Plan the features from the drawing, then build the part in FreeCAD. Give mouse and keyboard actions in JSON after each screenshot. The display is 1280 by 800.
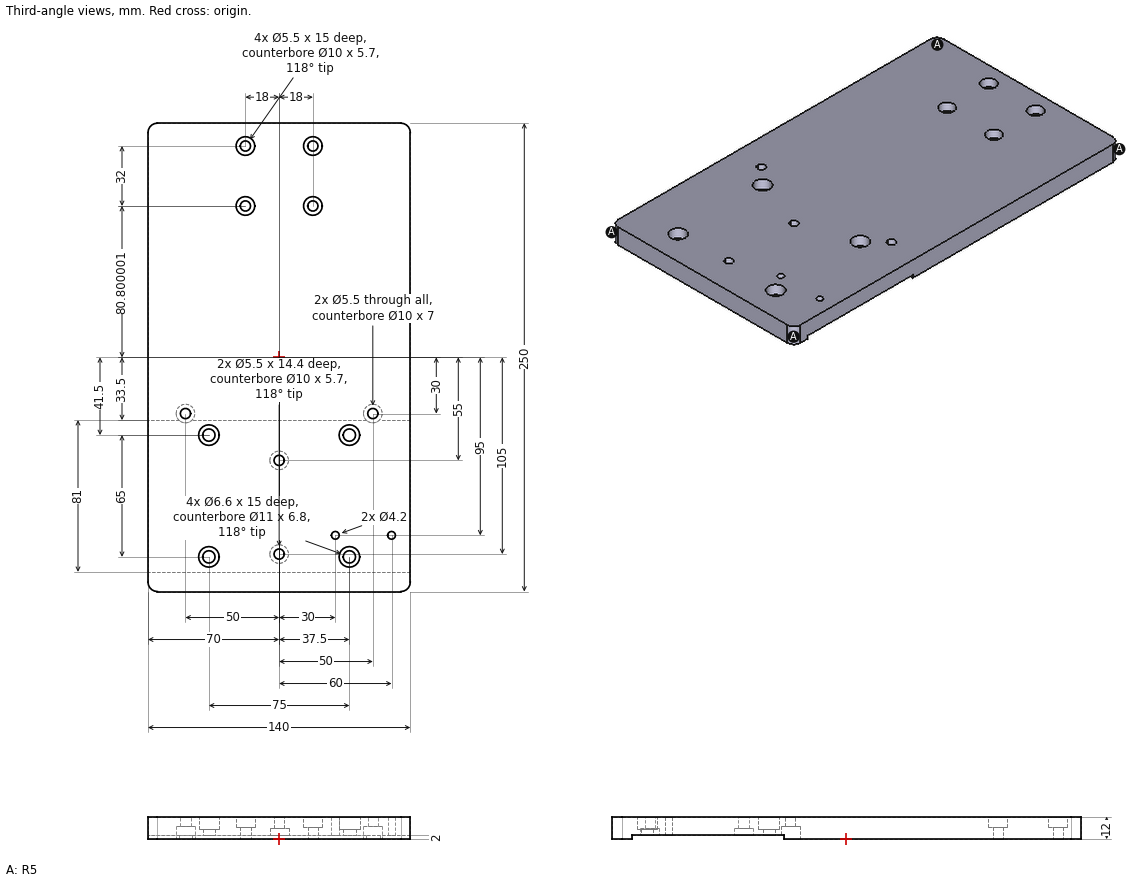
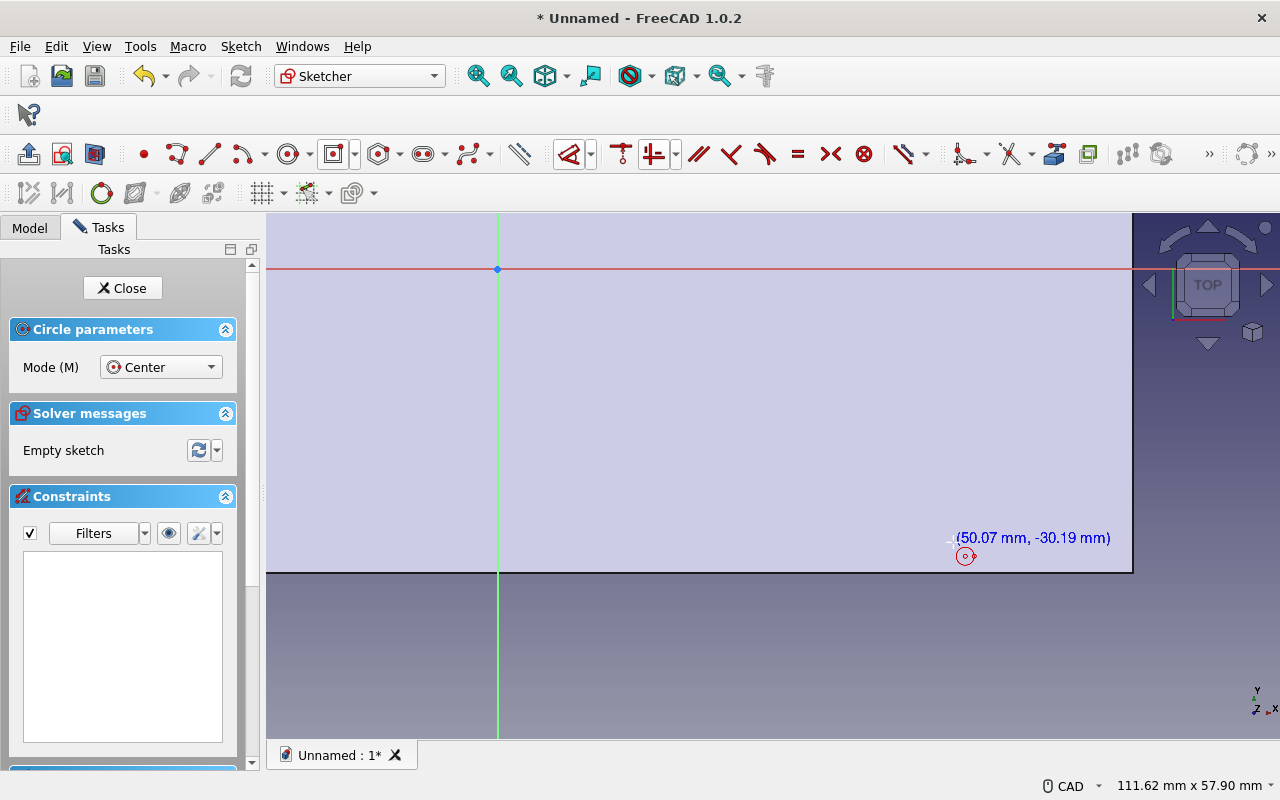
{"action": "left_click", "coordinate": [952, 542]}
{"action": "left_click", "coordinate": [969, 524]}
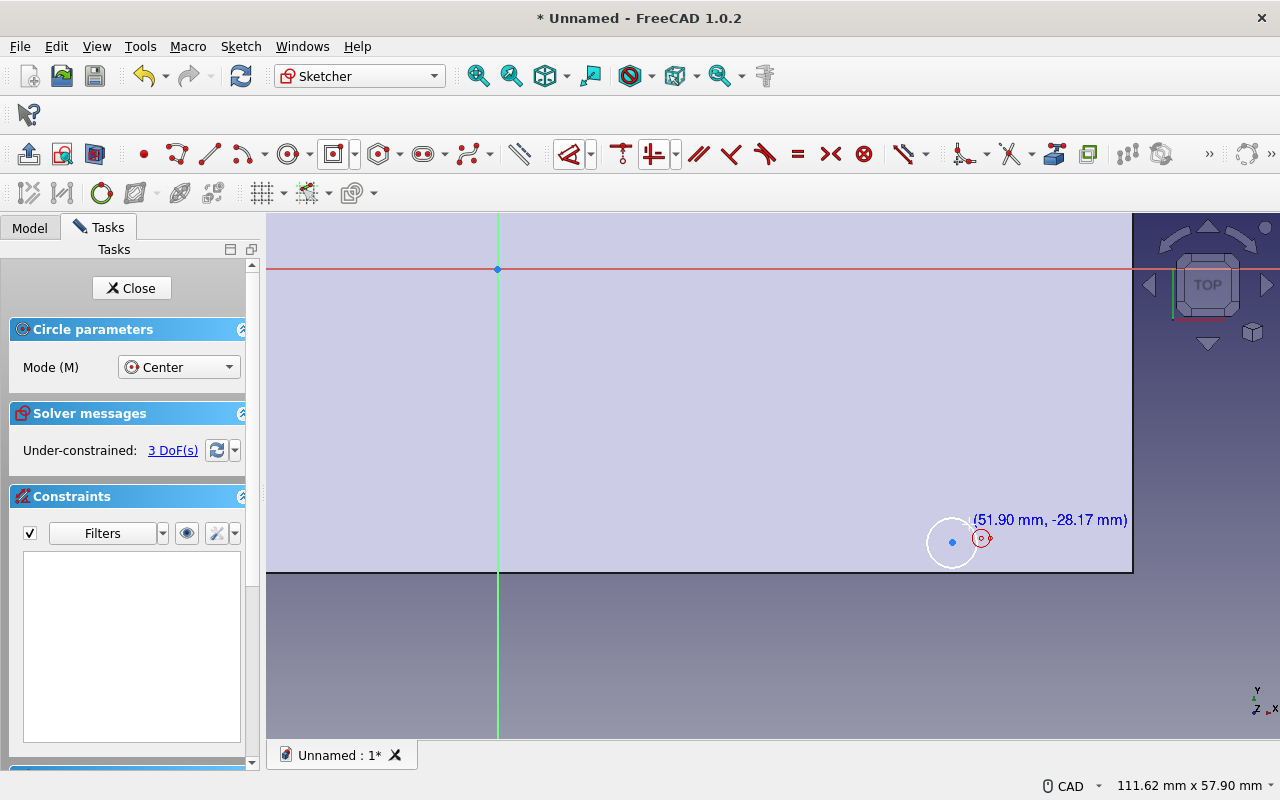
{"action": "scroll", "coordinate": [956, 547], "scroll_direction": "down", "scroll_amount": 3}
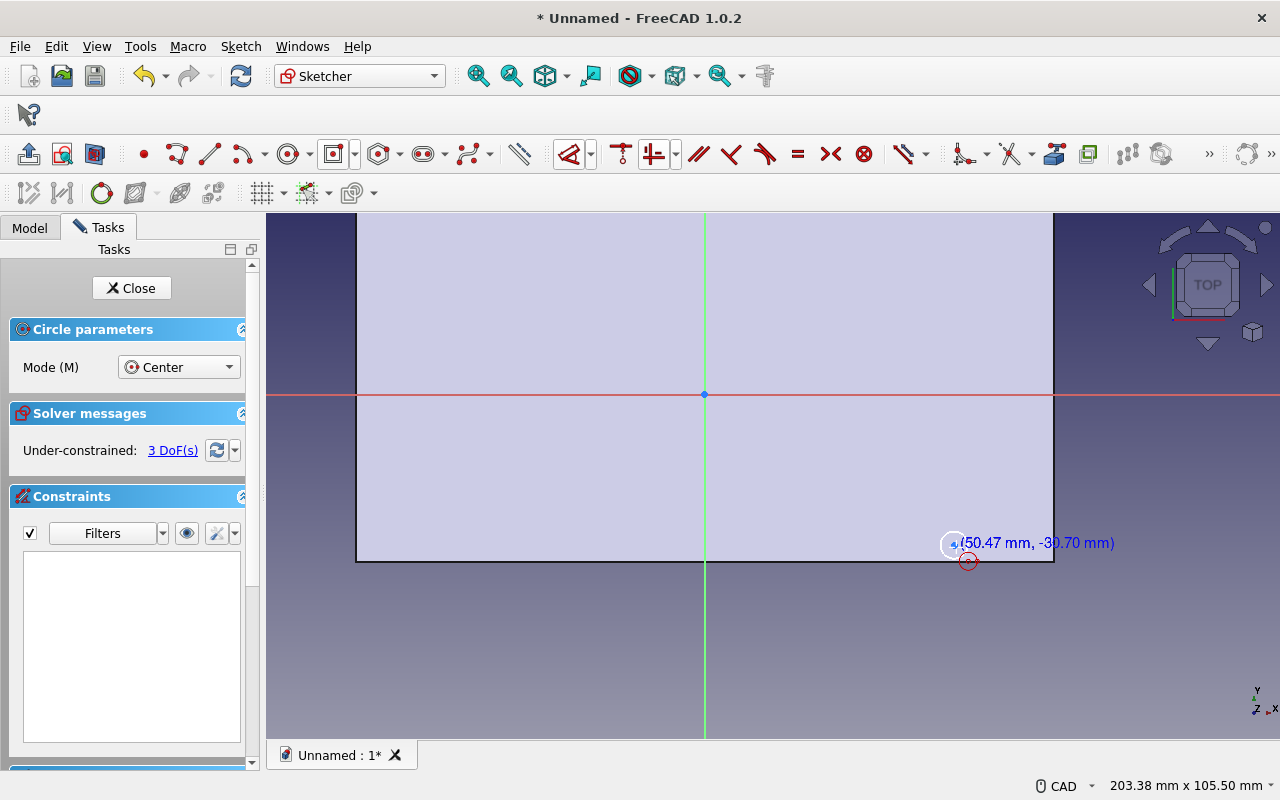
{"action": "scroll", "coordinate": [455, 544], "scroll_direction": "up", "scroll_amount": 3}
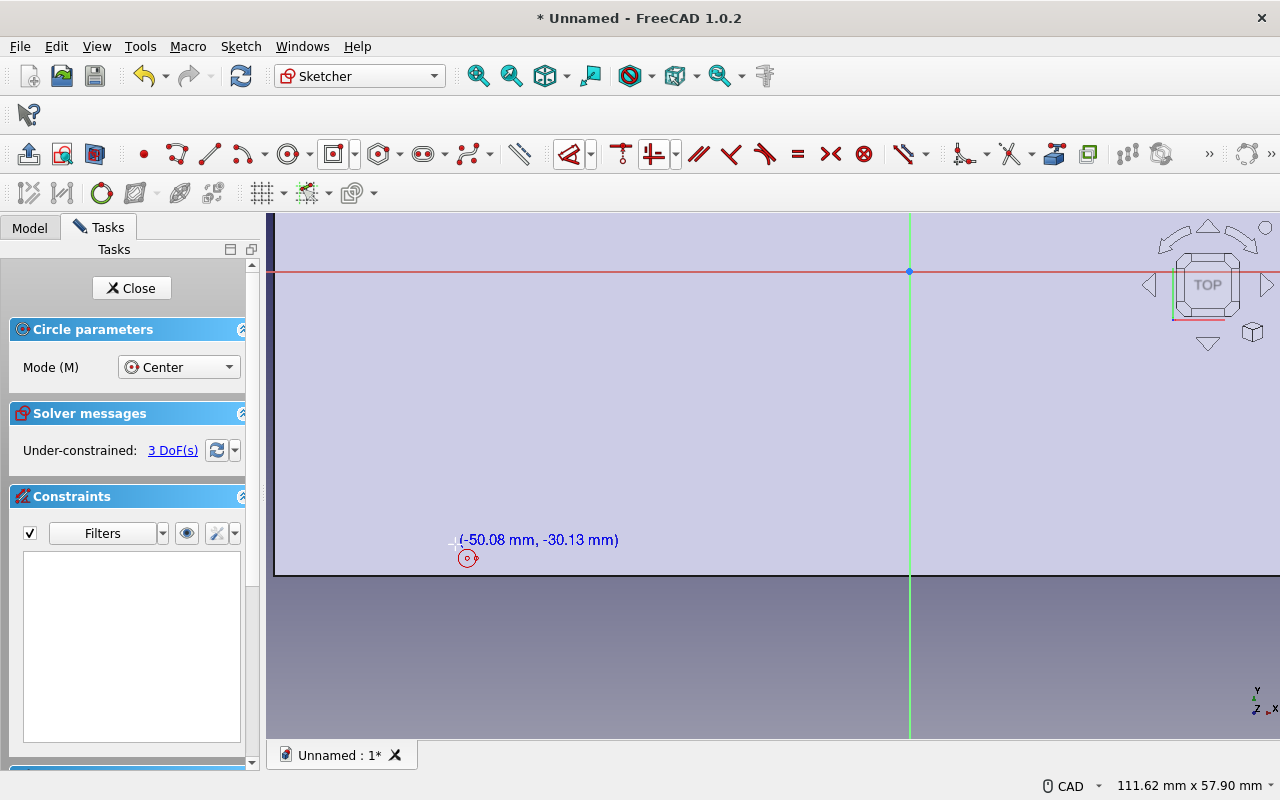
{"action": "left_click", "coordinate": [456, 544]}
{"action": "left_click", "coordinate": [473, 526]}
{"action": "key", "text": "Escape"}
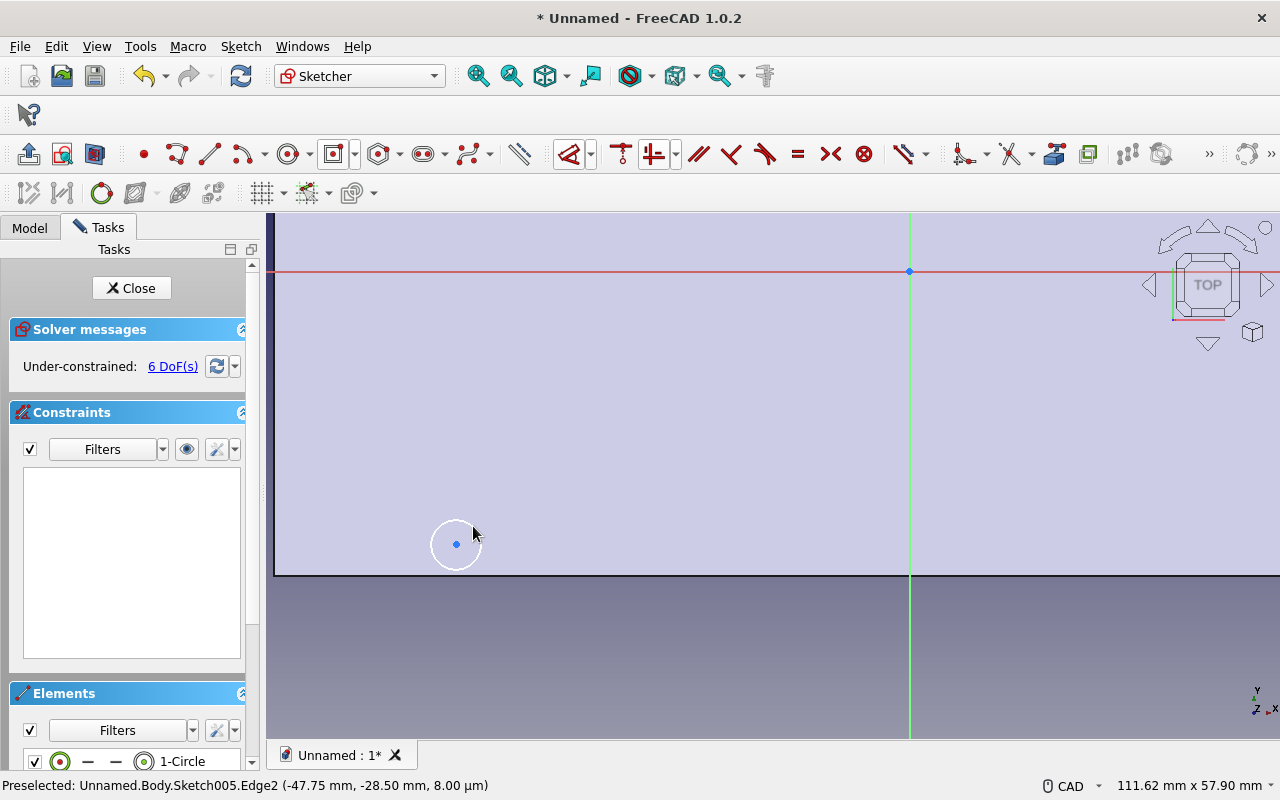
{"action": "scroll", "coordinate": [455, 544], "scroll_direction": "down", "scroll_amount": 3}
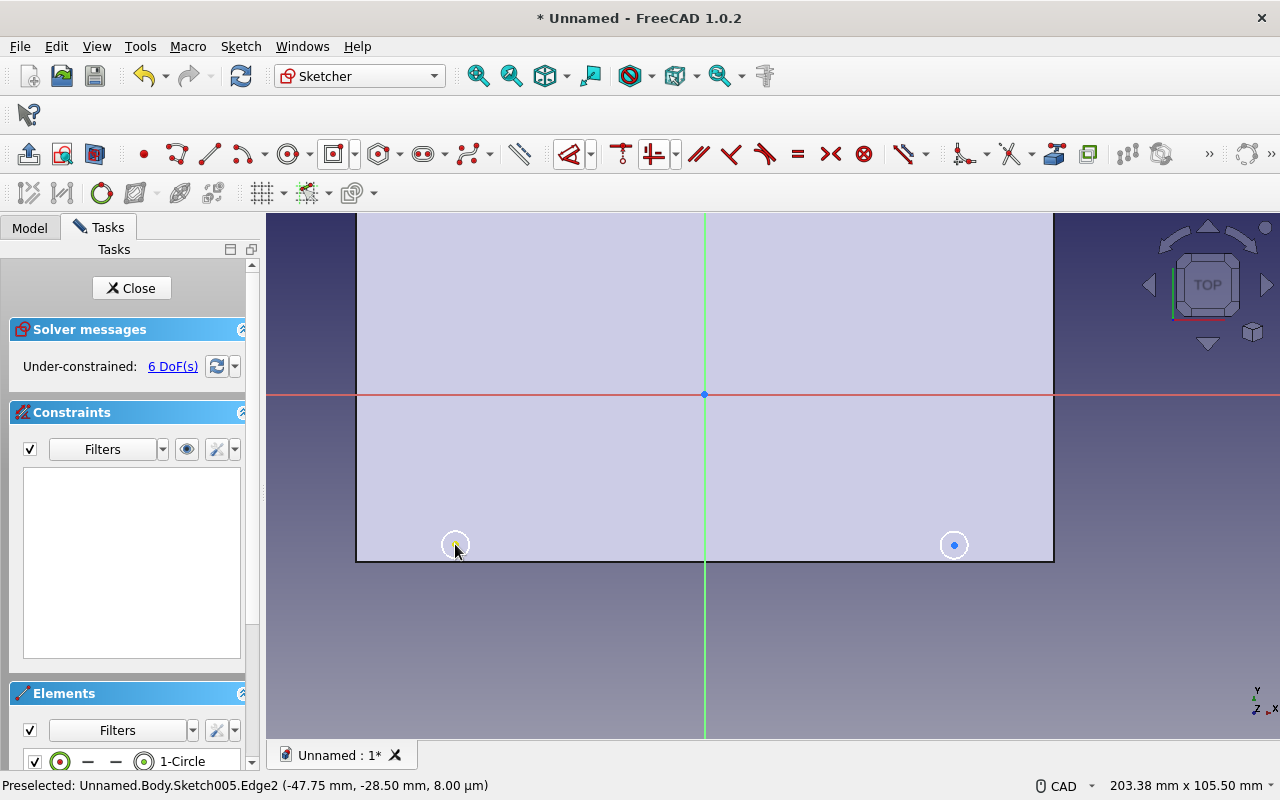
{"action": "left_click", "coordinate": [964, 535]}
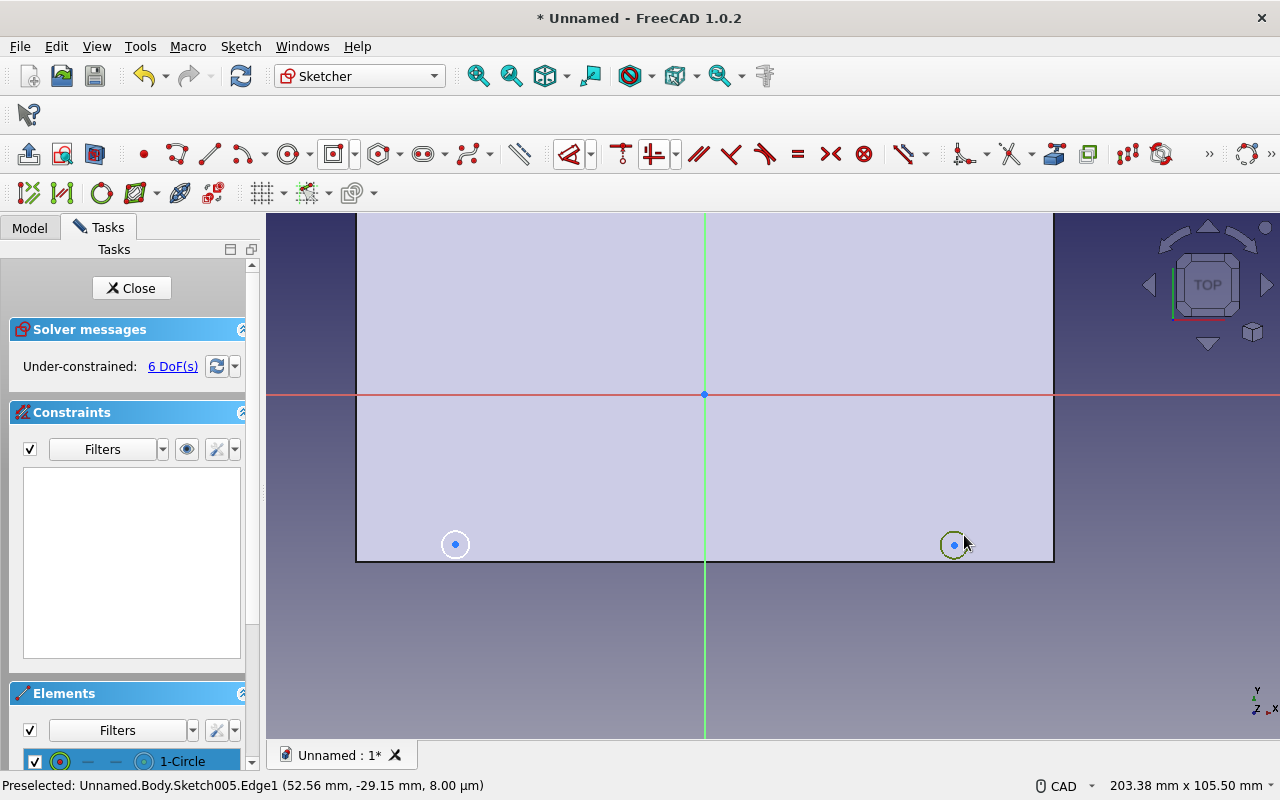
{"action": "left_click", "coordinate": [465, 535]}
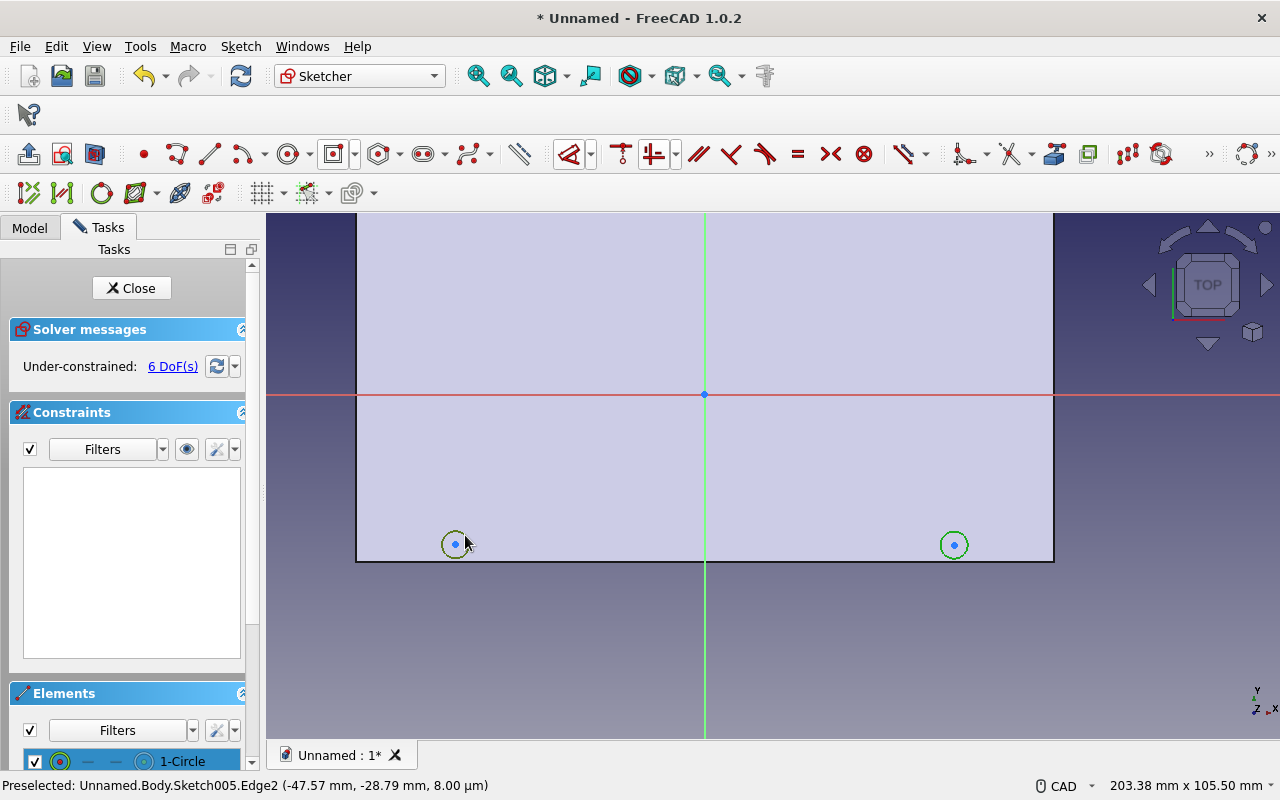
{"action": "left_click", "coordinate": [798, 154]}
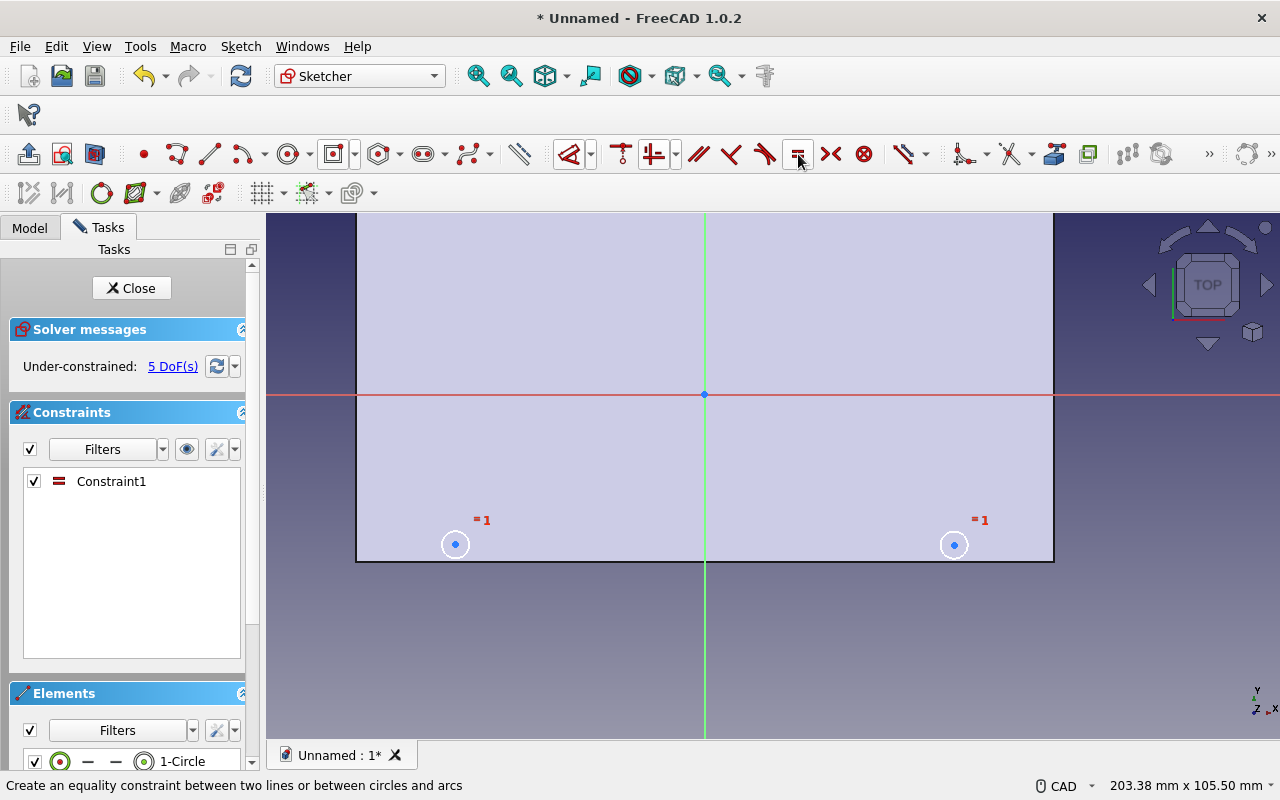
{"action": "left_click", "coordinate": [954, 545]}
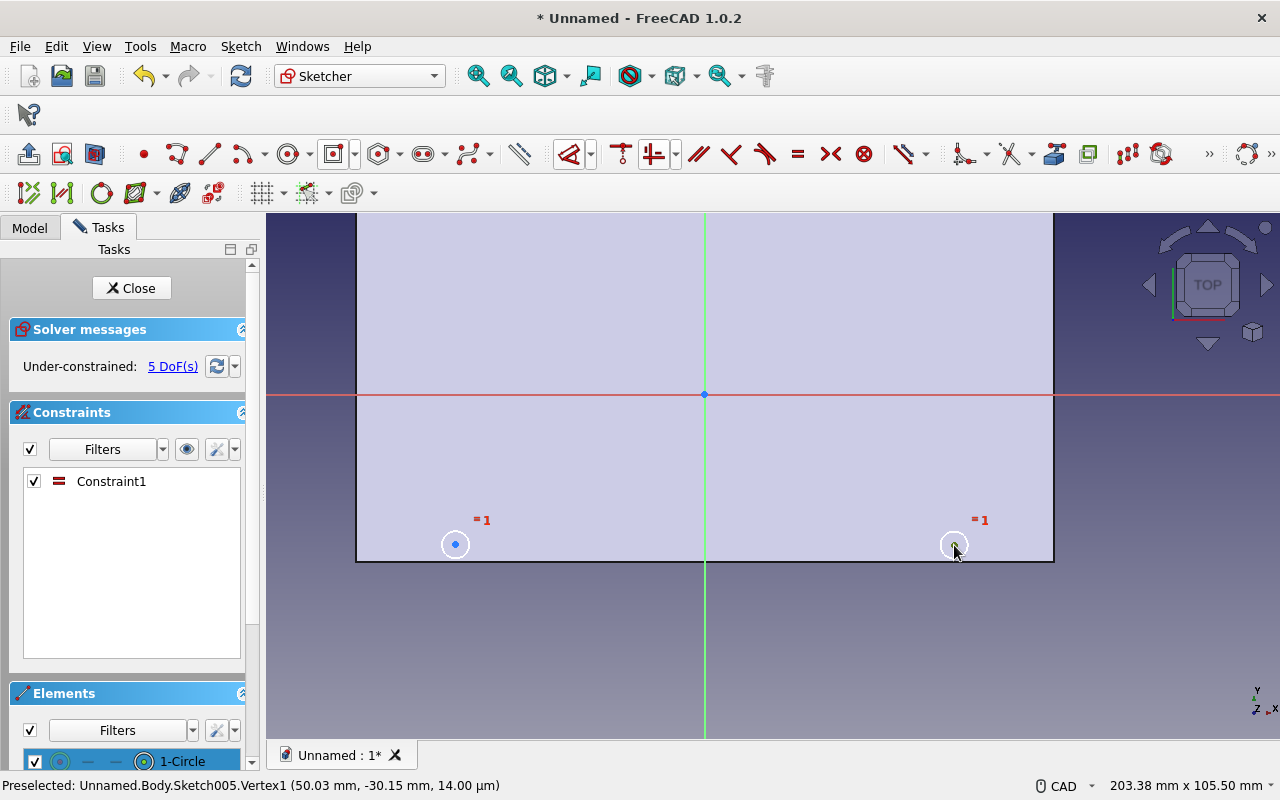
{"action": "left_click", "coordinate": [456, 545]}